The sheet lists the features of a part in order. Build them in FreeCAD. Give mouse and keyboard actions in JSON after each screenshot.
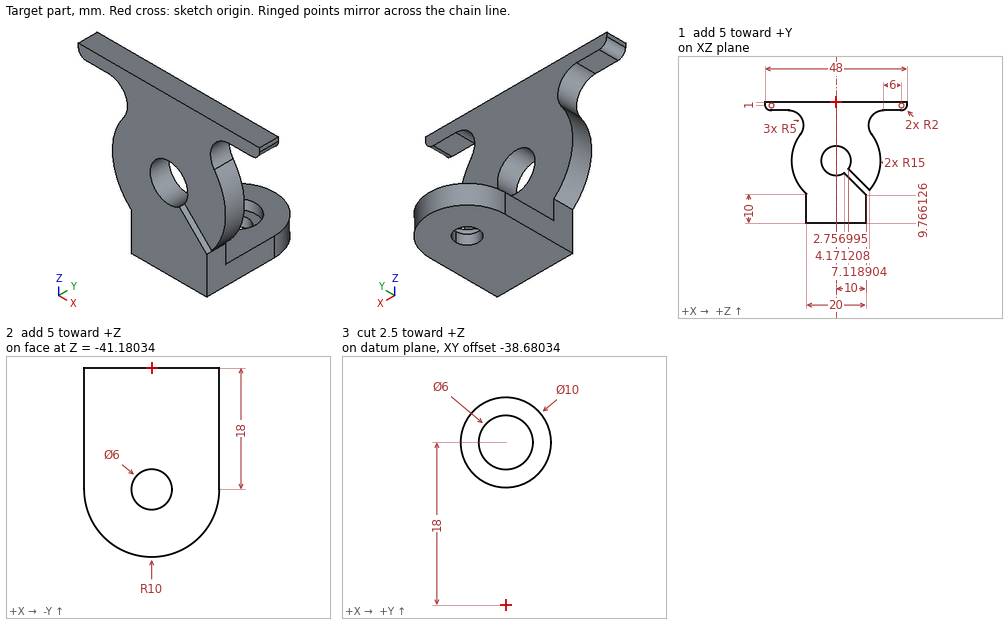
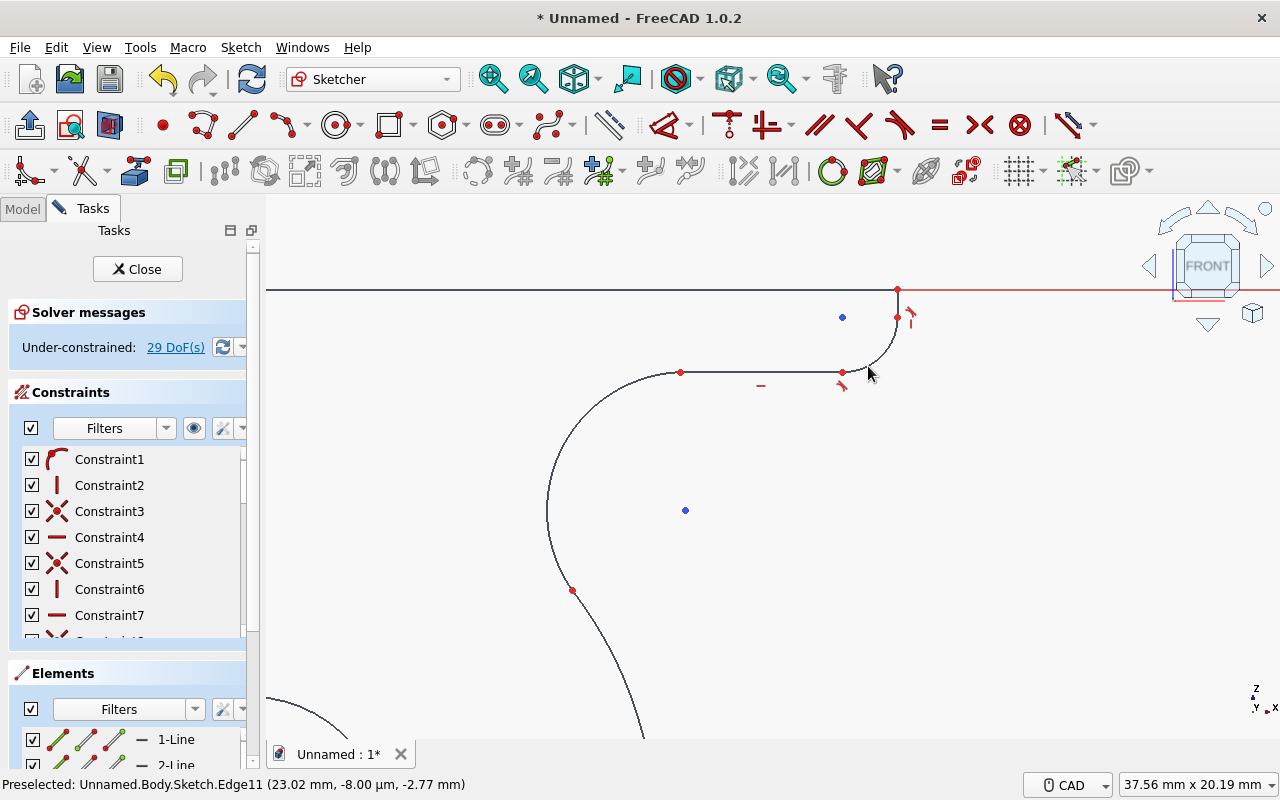
{"action": "left_click", "coordinate": [794, 372]}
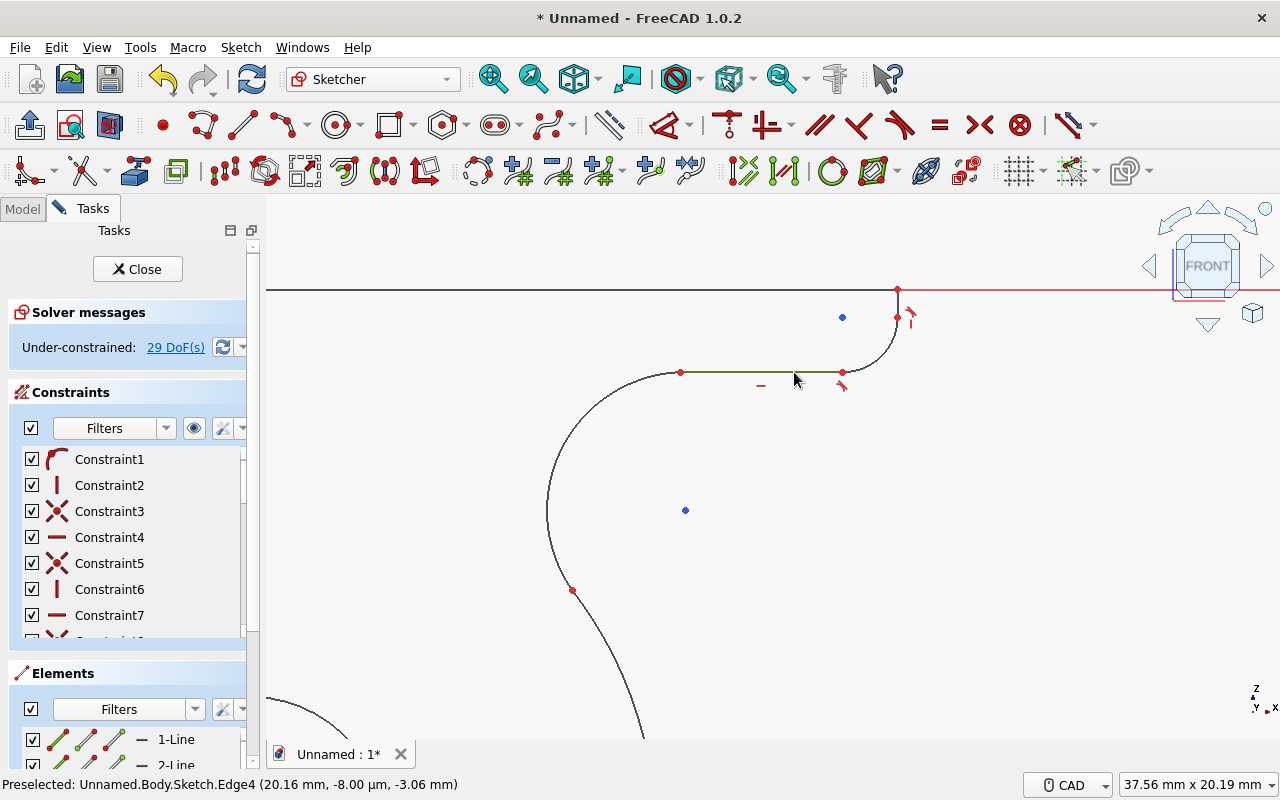
{"action": "left_click", "coordinate": [599, 403]}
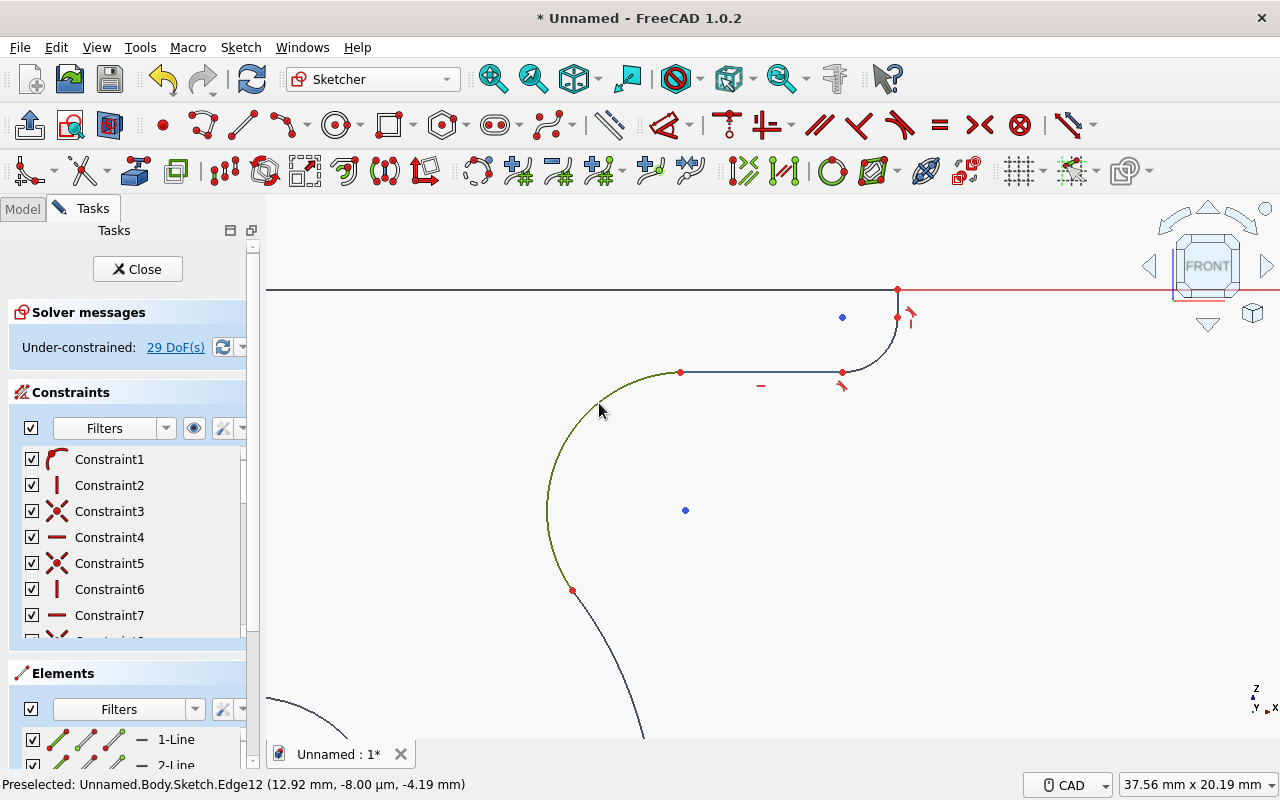
{"action": "left_click", "coordinate": [900, 126]}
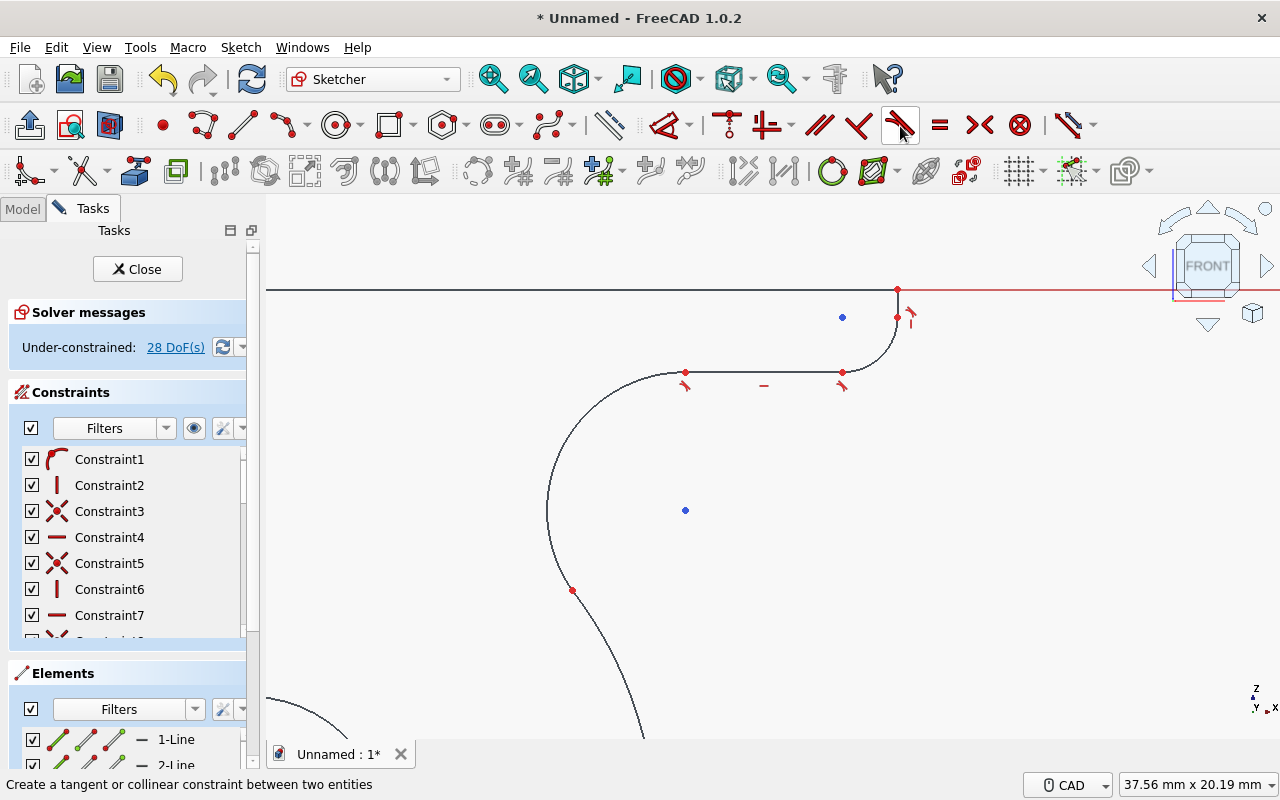
{"action": "scroll", "coordinate": [901, 303], "scroll_direction": "down", "scroll_amount": 6}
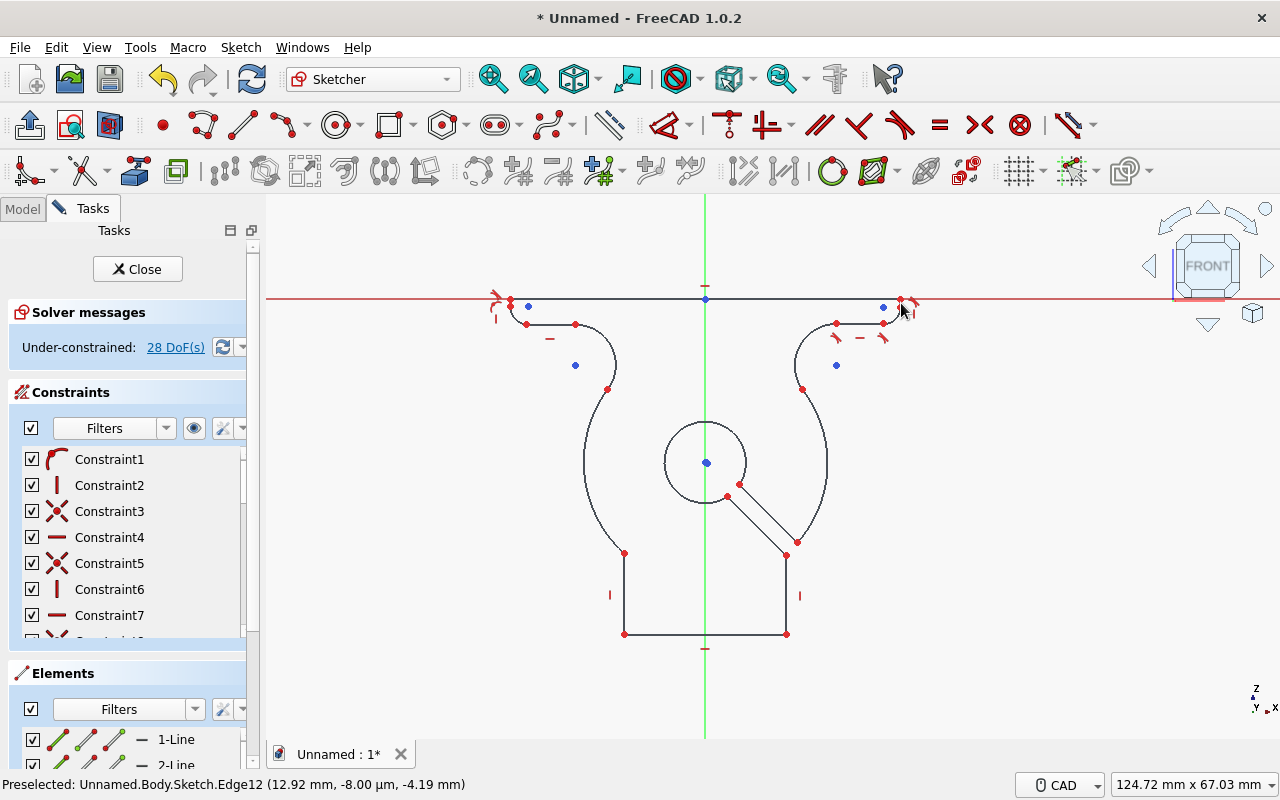
{"action": "left_click", "coordinate": [561, 325]}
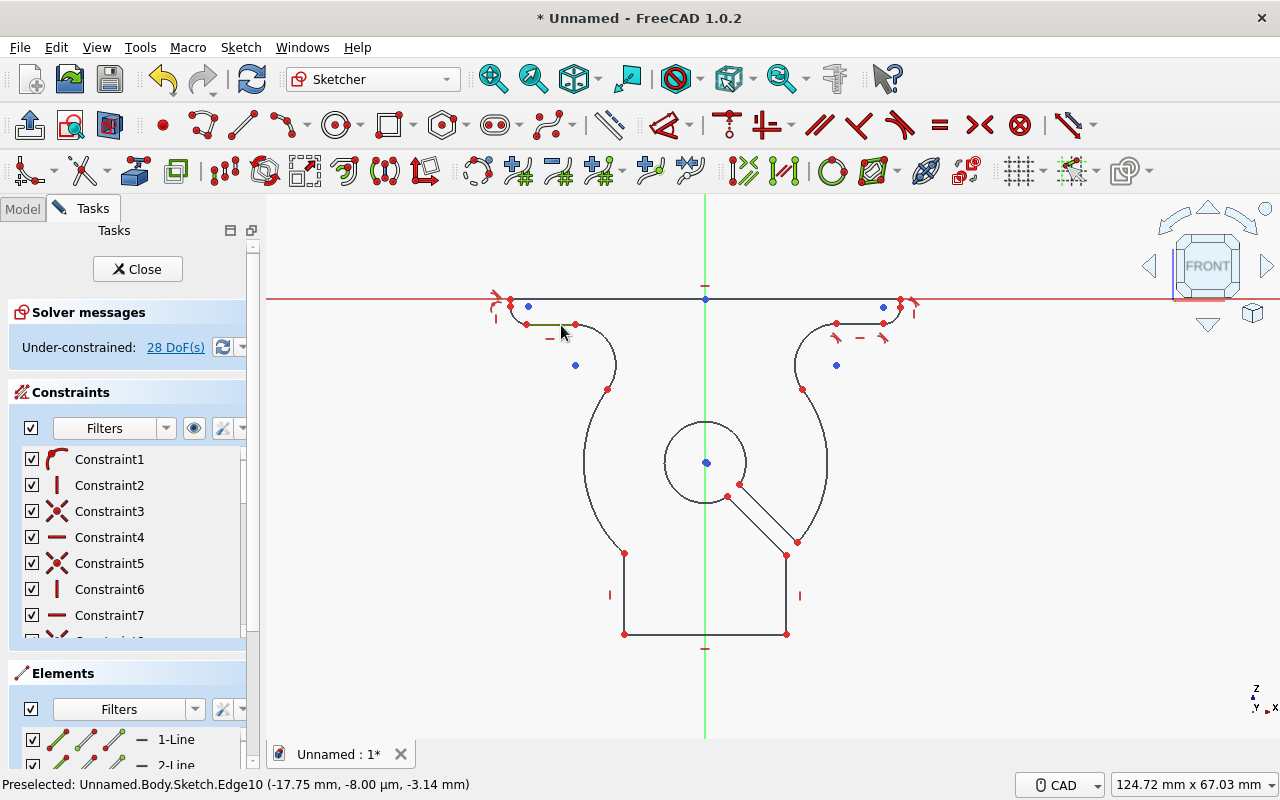
{"action": "left_click", "coordinate": [616, 365]}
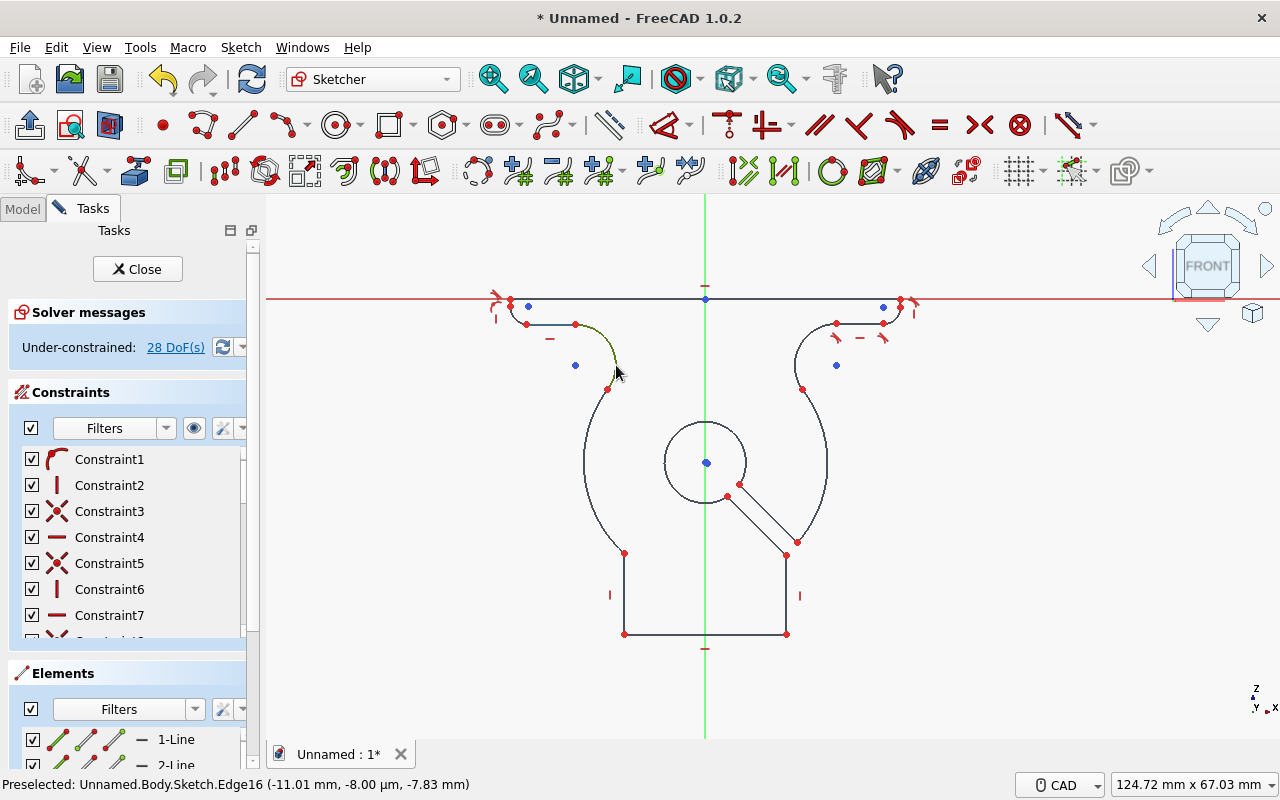
{"action": "left_click", "coordinate": [900, 126]}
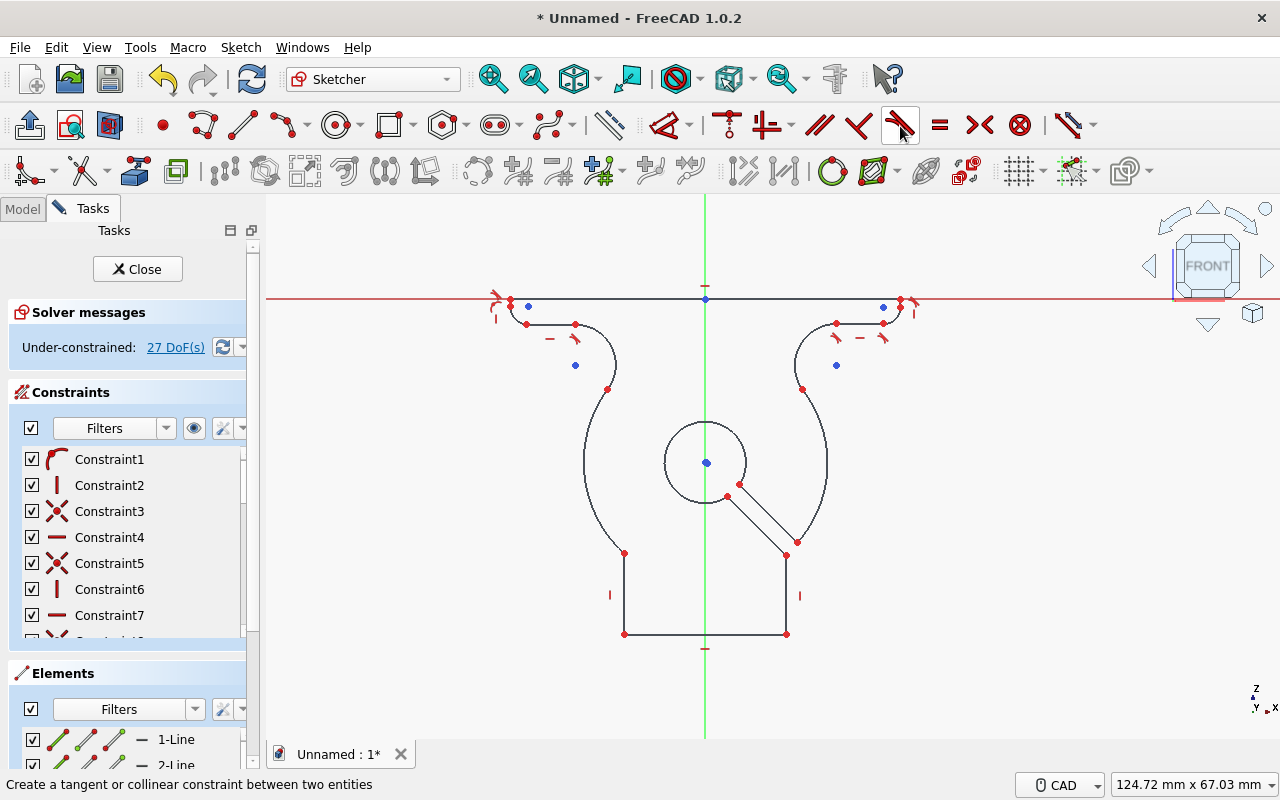
{"action": "left_click", "coordinate": [561, 325]}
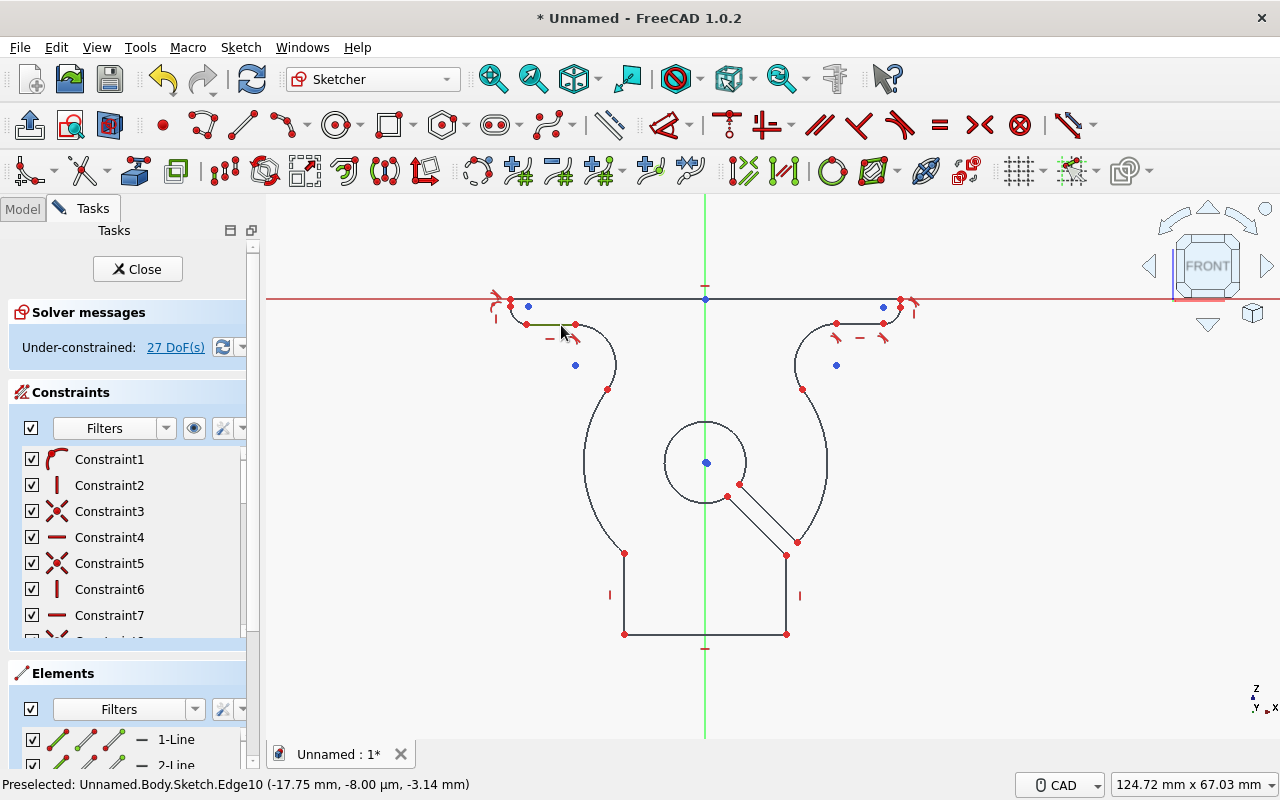
{"action": "left_click", "coordinate": [515, 319]}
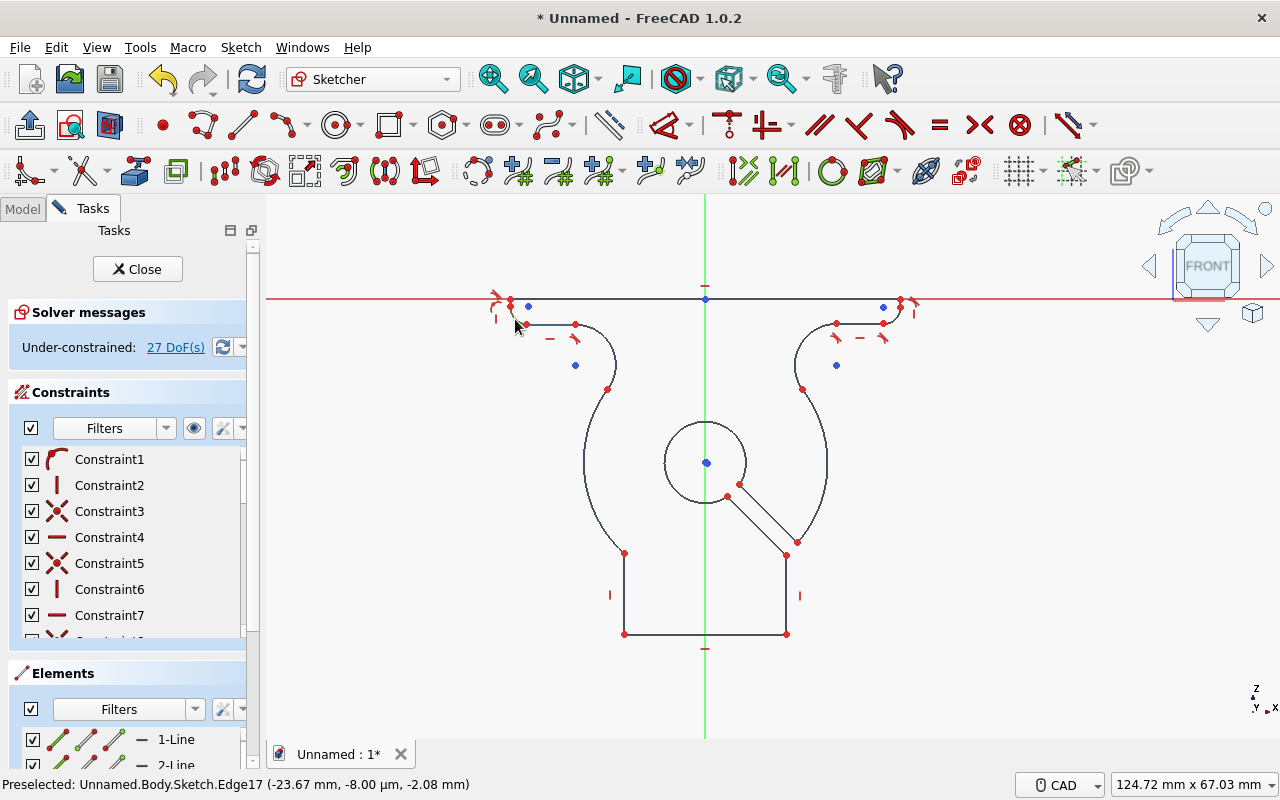
{"action": "key", "text": "t"}